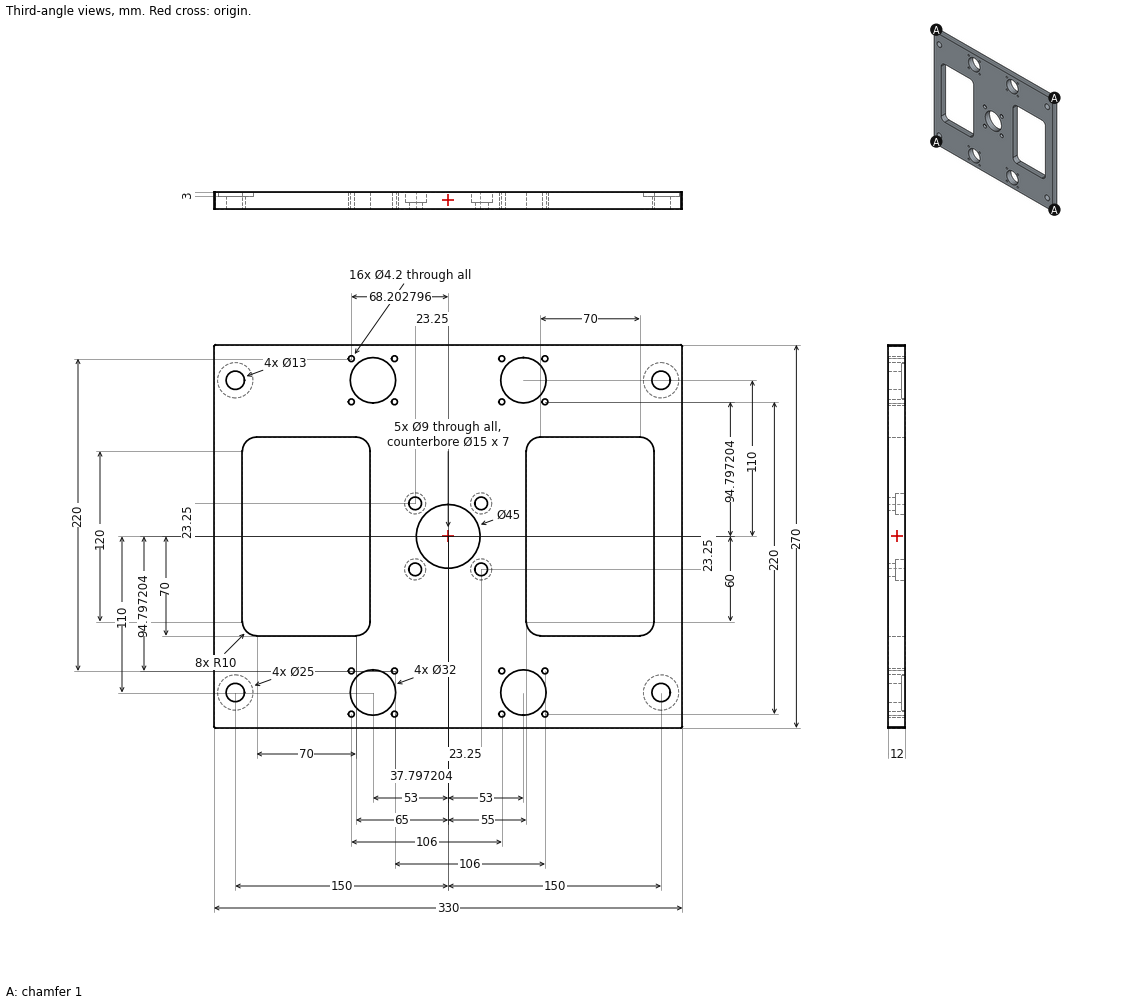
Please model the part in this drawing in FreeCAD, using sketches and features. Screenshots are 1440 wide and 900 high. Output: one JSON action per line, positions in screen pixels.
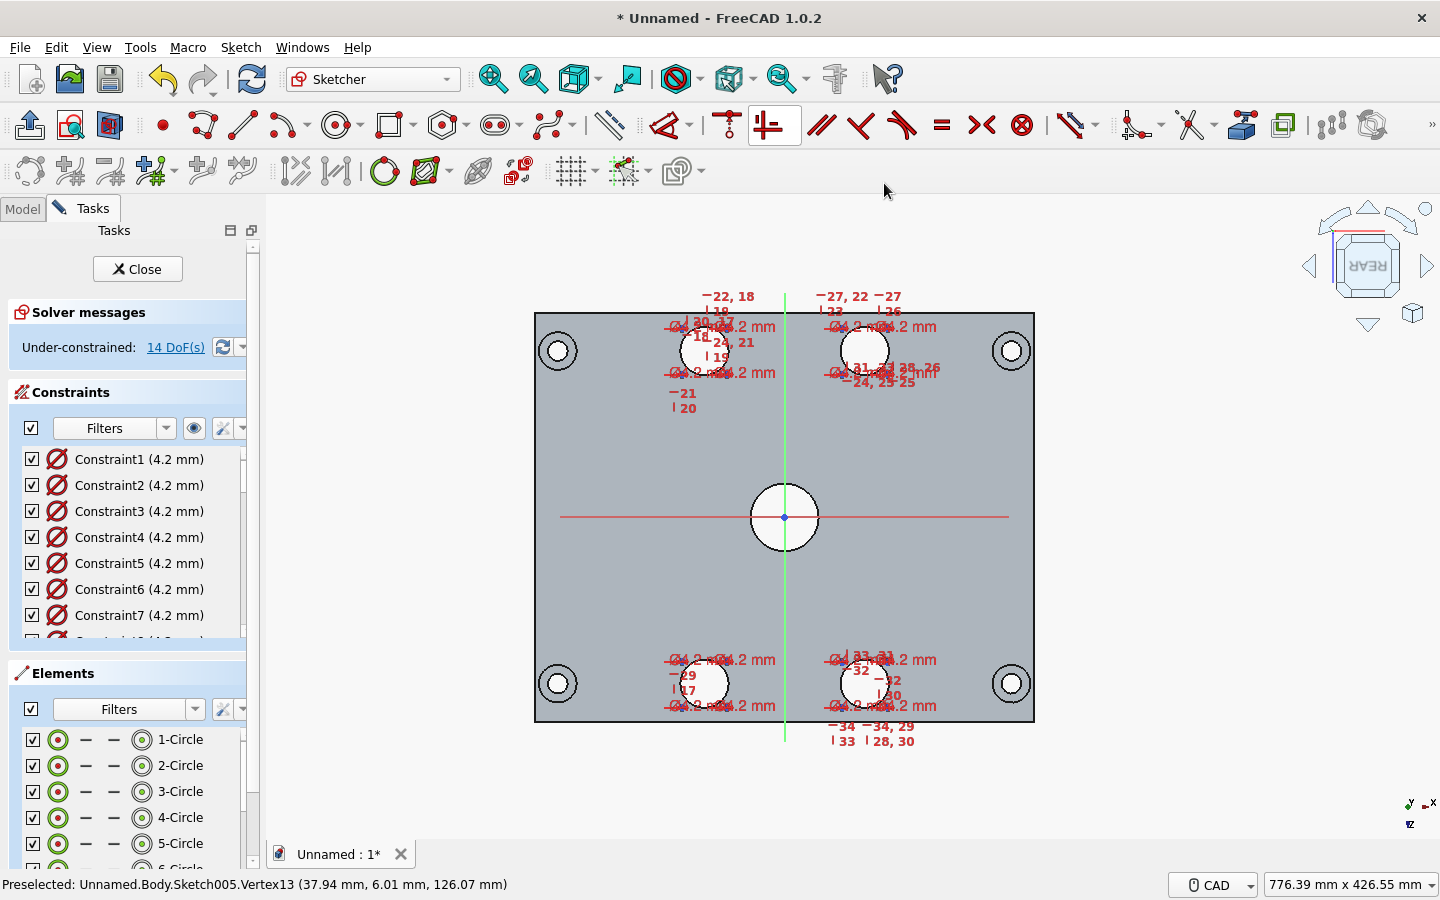
{"action": "left_click", "coordinate": [727, 375]}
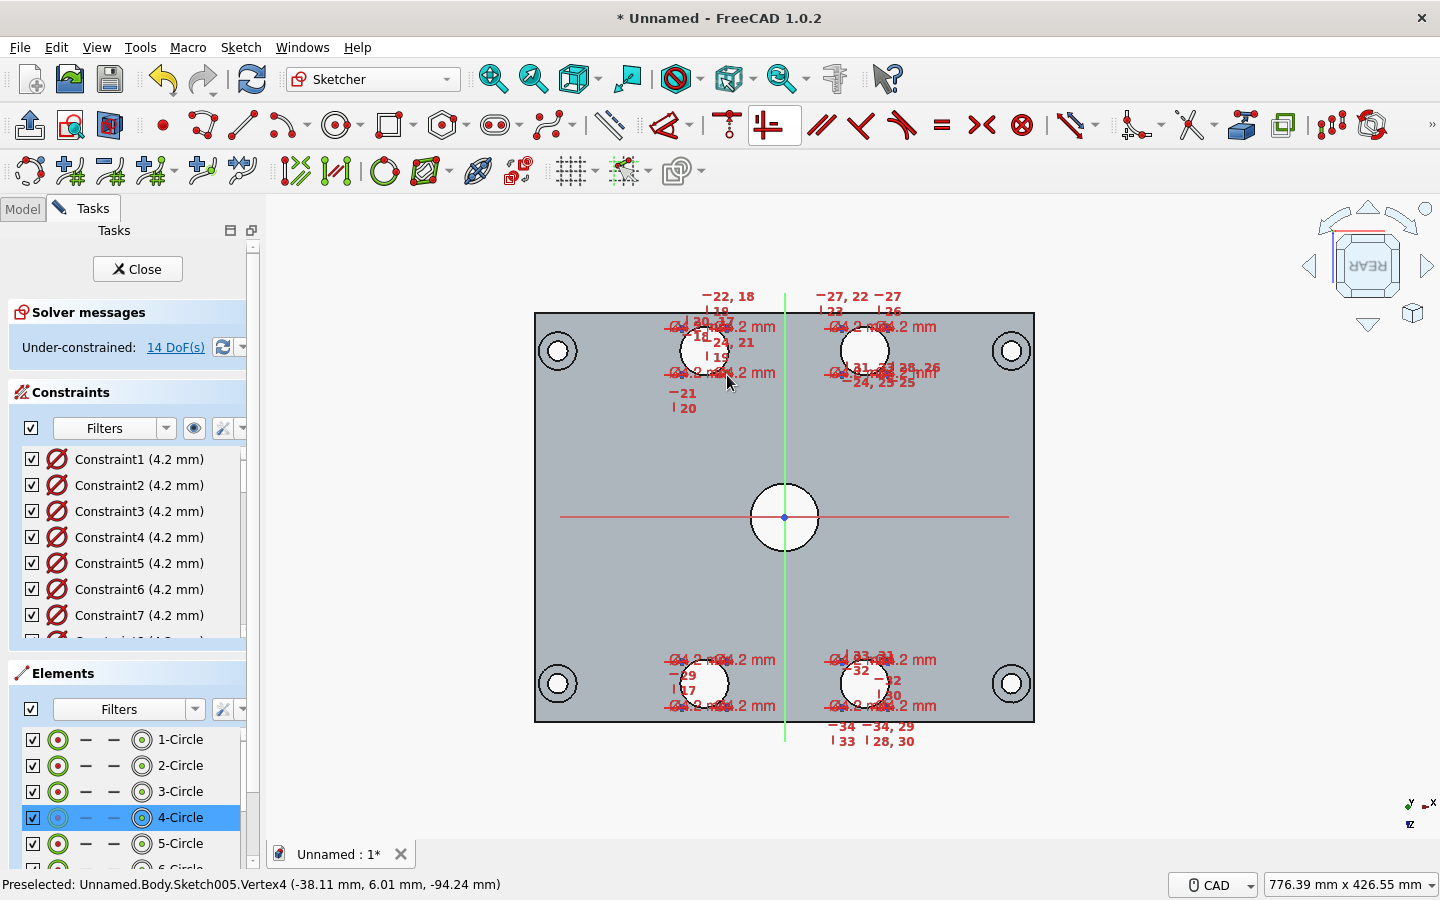
{"action": "left_click", "coordinate": [727, 708]}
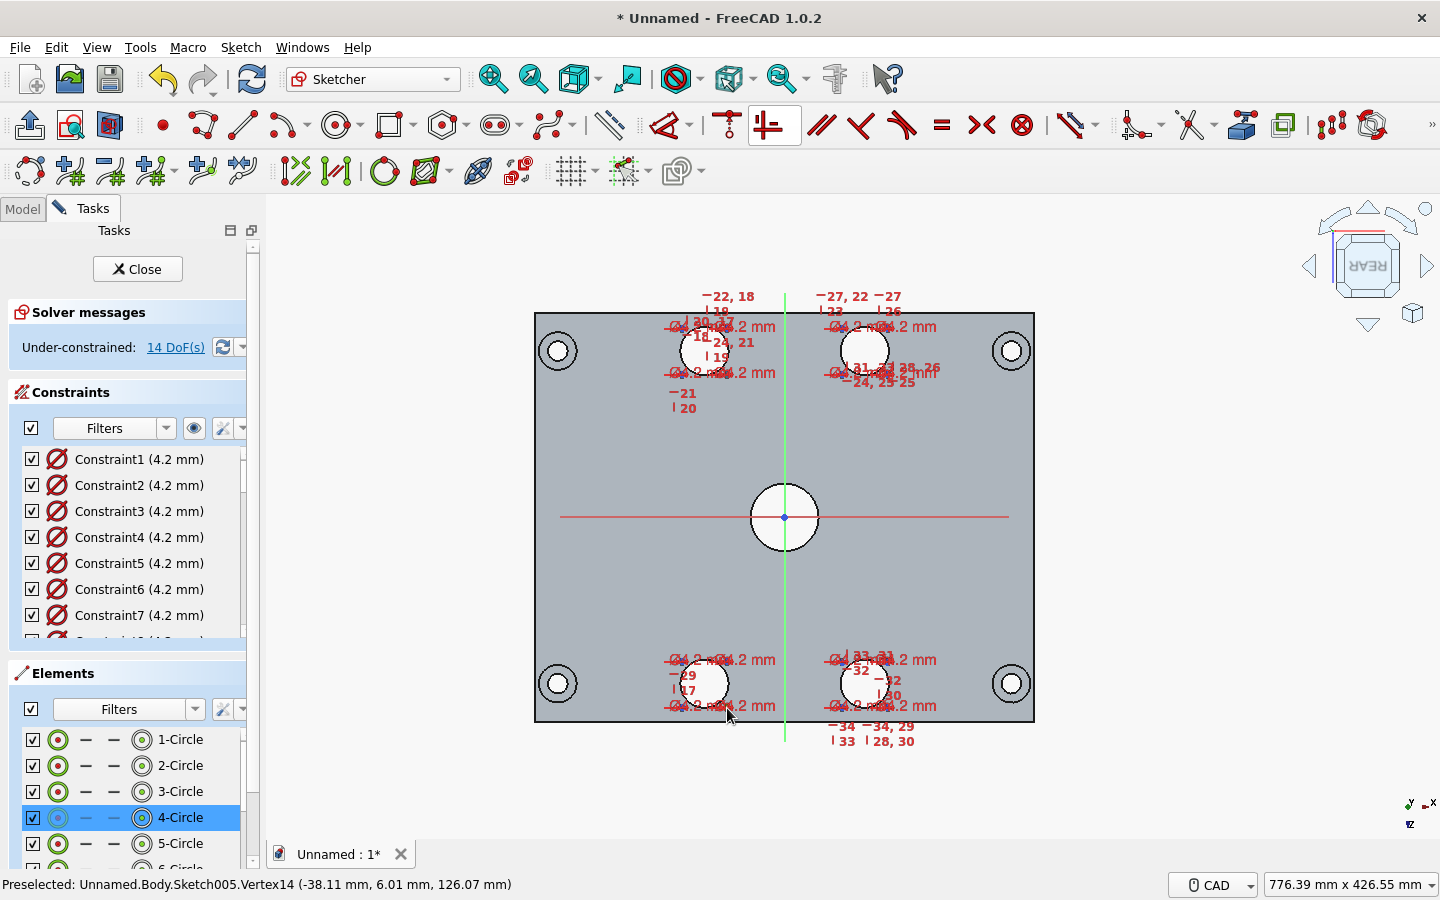
{"action": "key", "text": "v"}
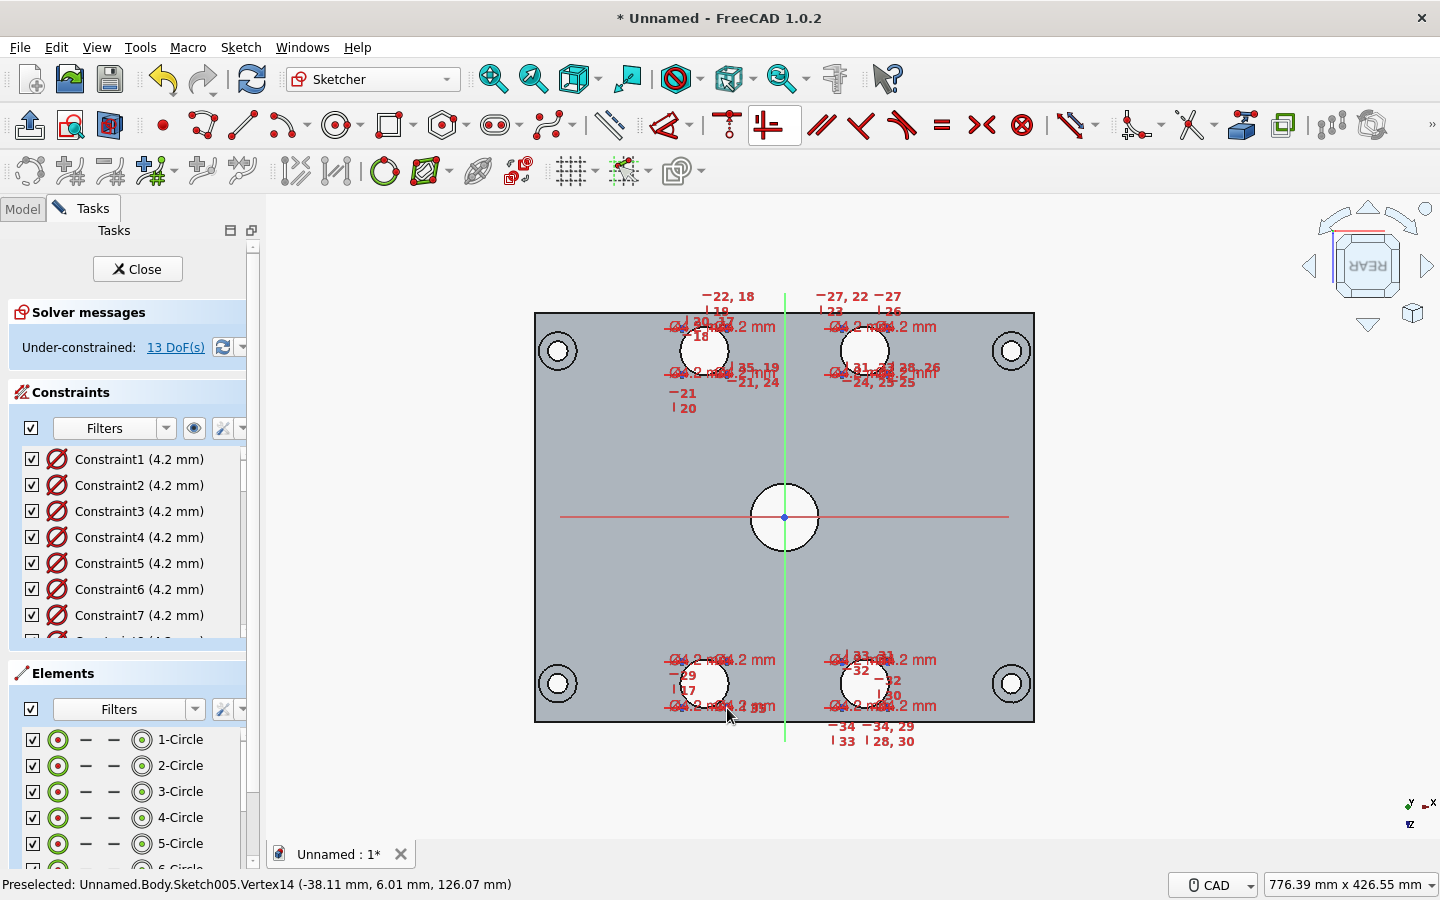
{"action": "left_click", "coordinate": [682, 708]}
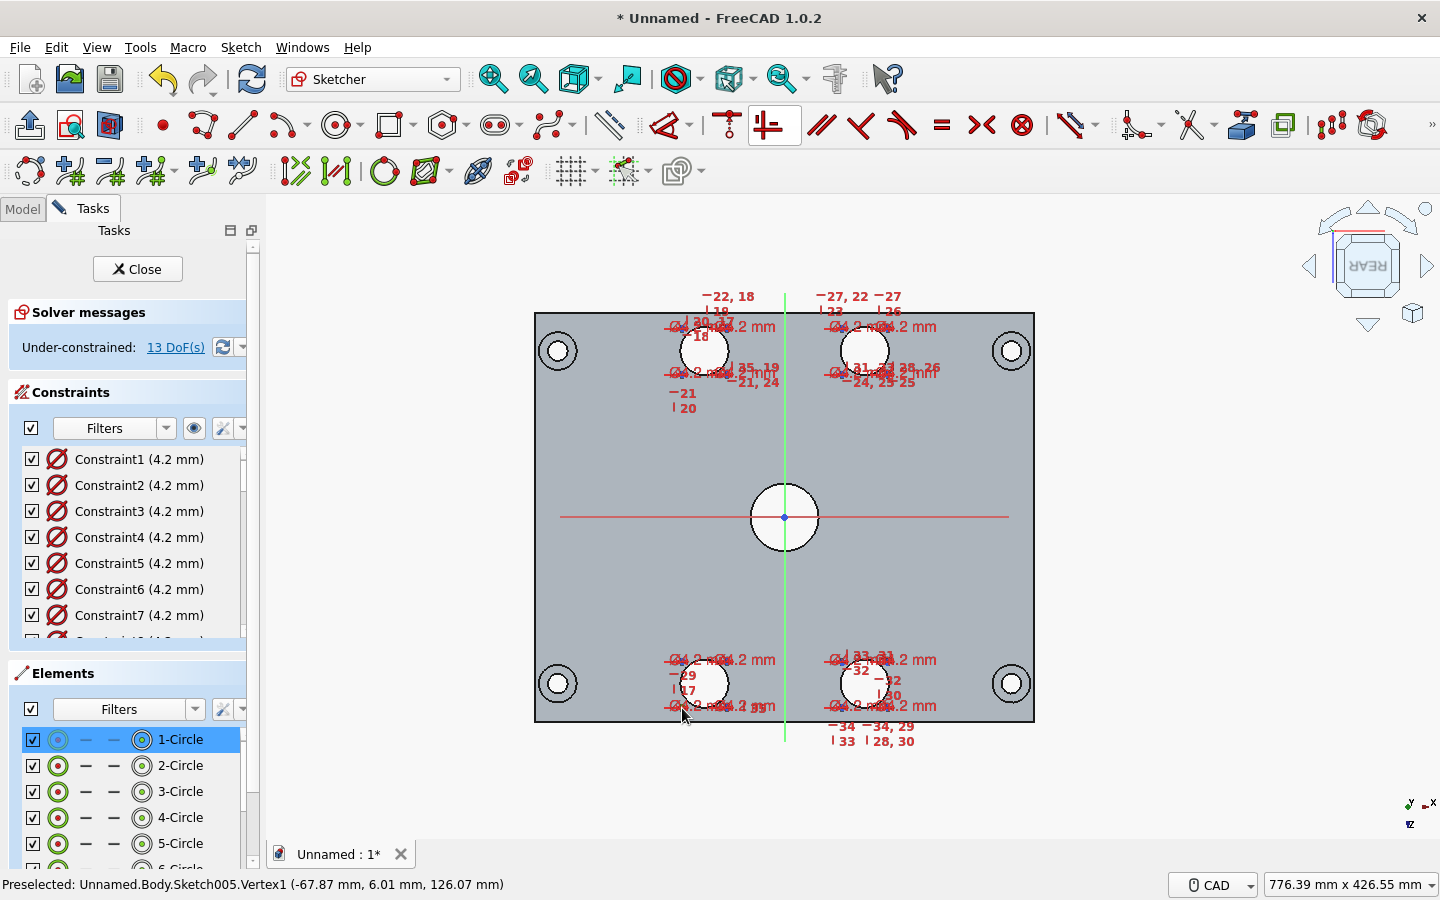
{"action": "left_click", "coordinate": [727, 708]}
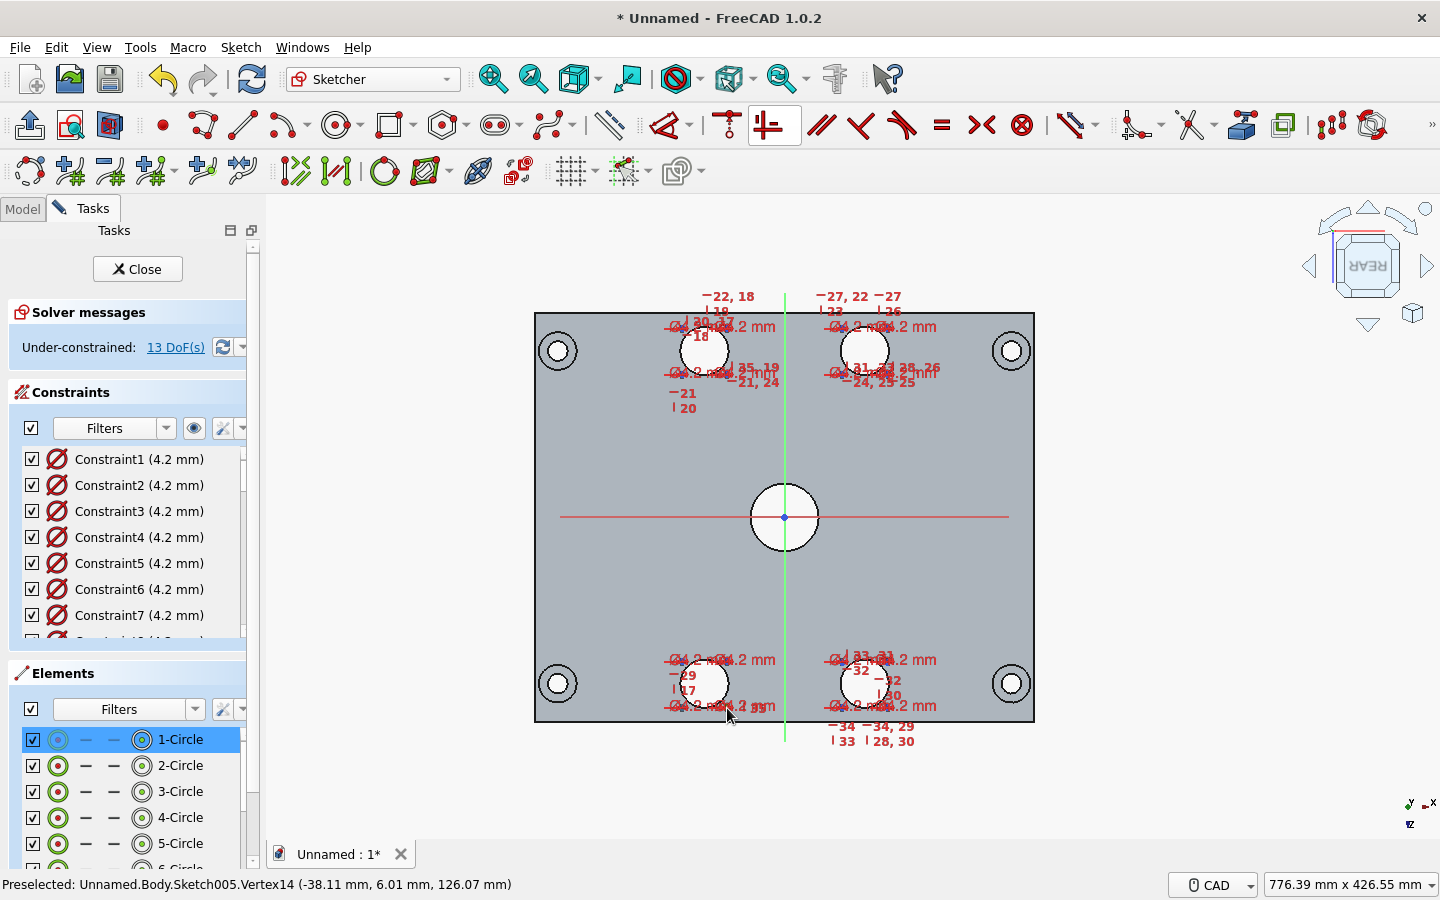
{"action": "left_click", "coordinate": [796, 126]}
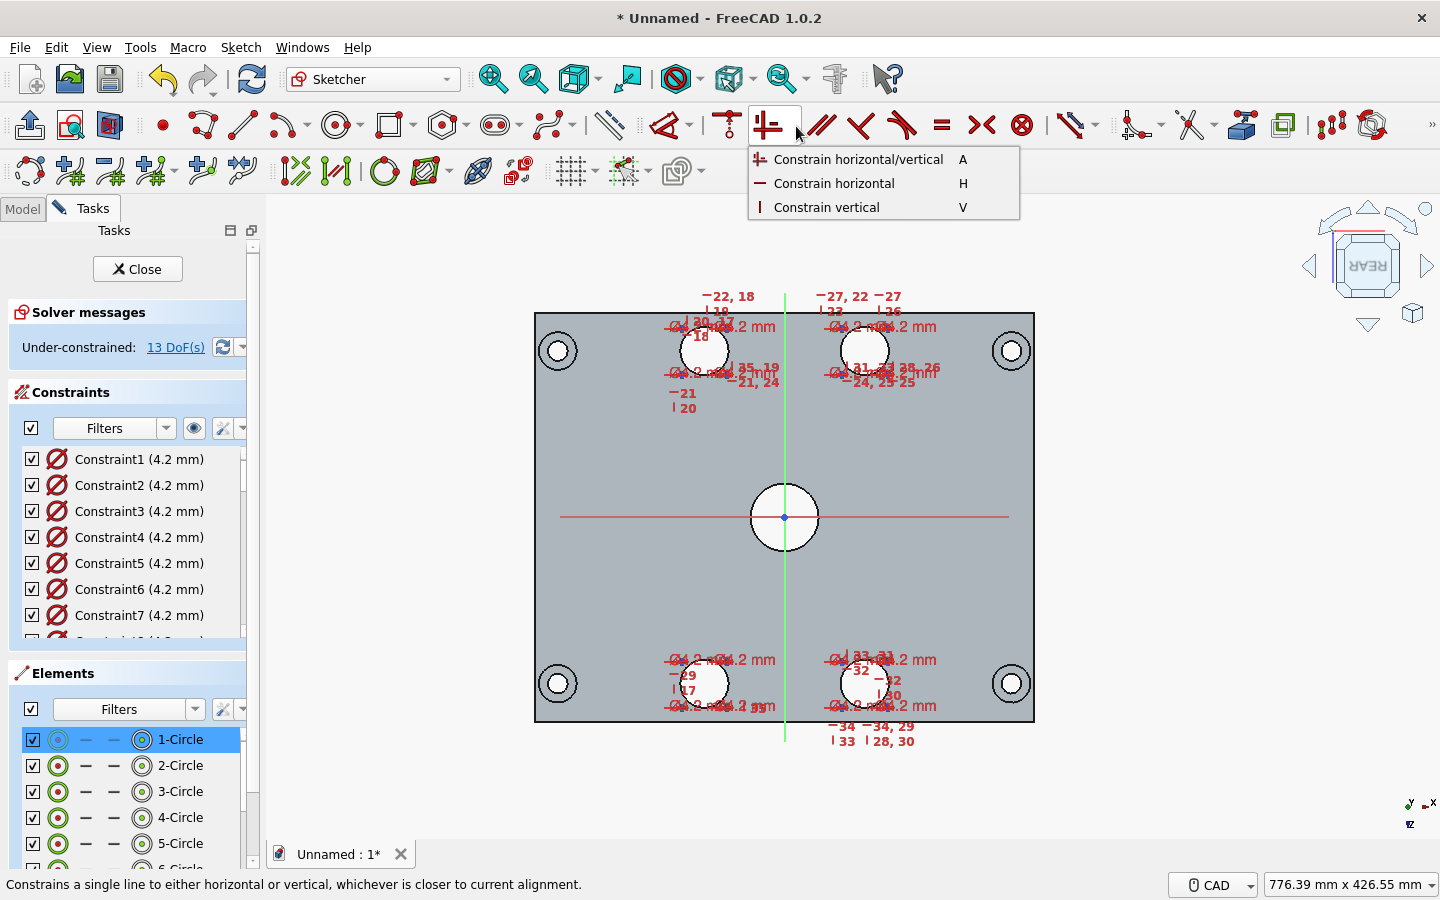
{"action": "left_click", "coordinate": [884, 183]}